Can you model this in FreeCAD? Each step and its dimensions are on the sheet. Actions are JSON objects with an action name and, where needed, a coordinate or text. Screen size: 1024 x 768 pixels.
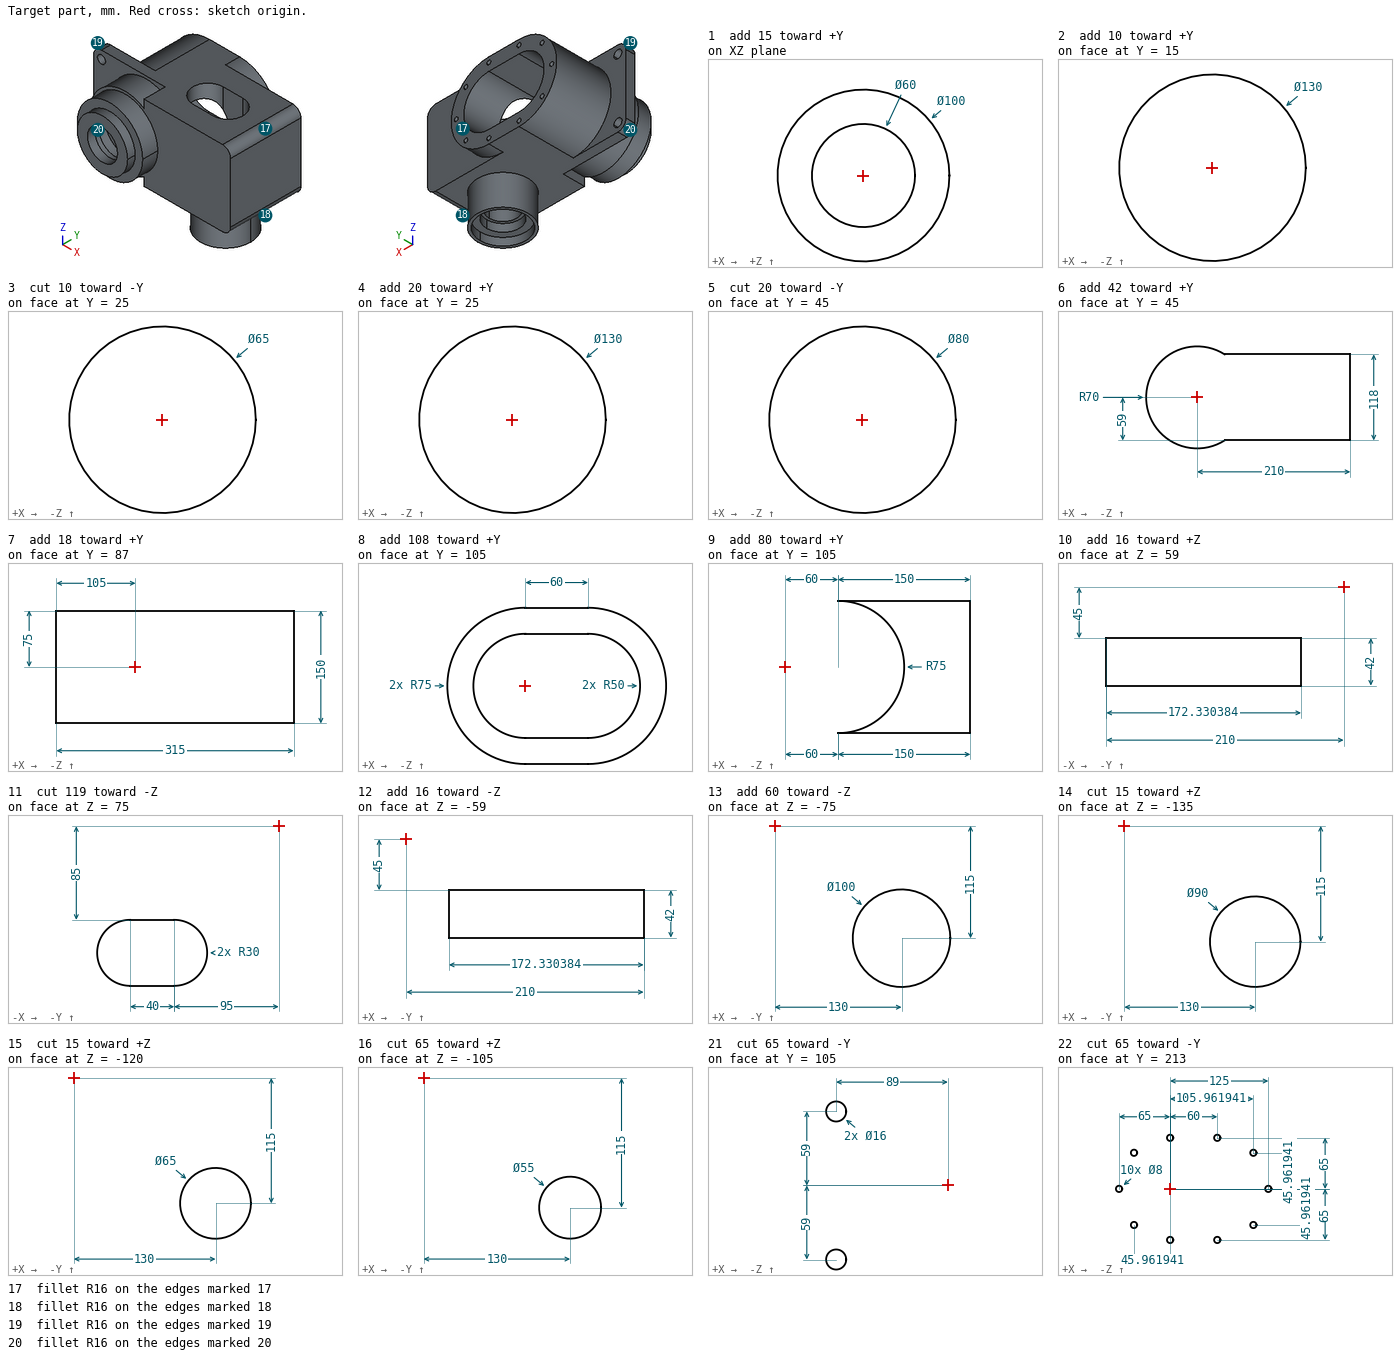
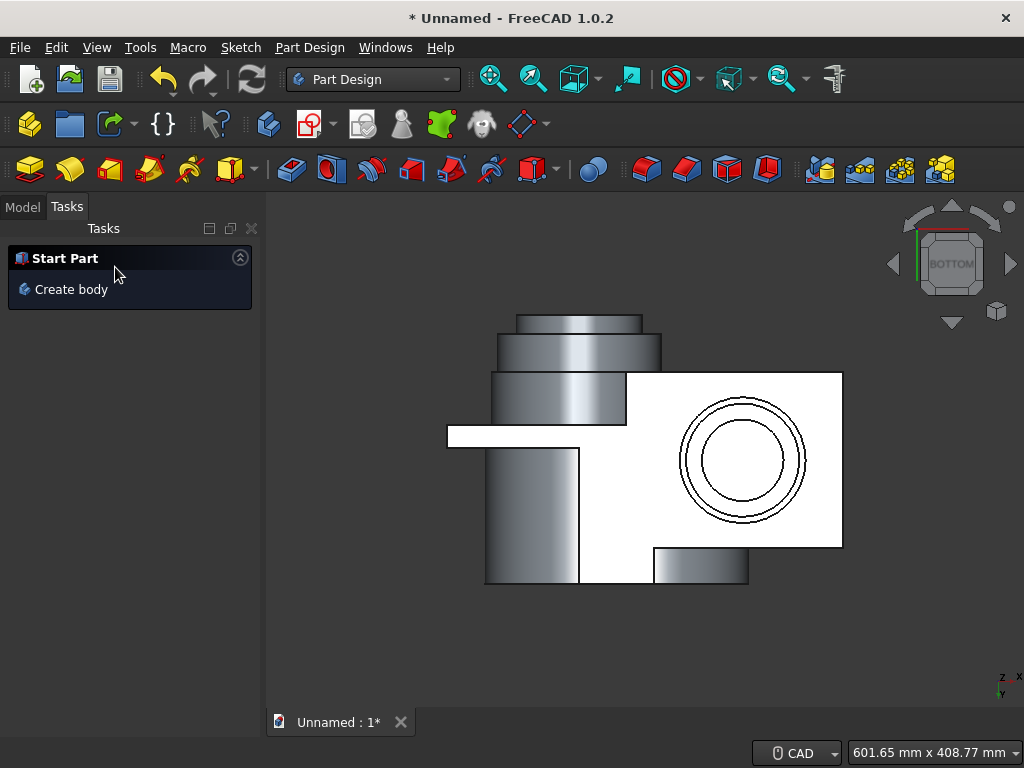
{"action": "left_click", "coordinate": [743, 459]}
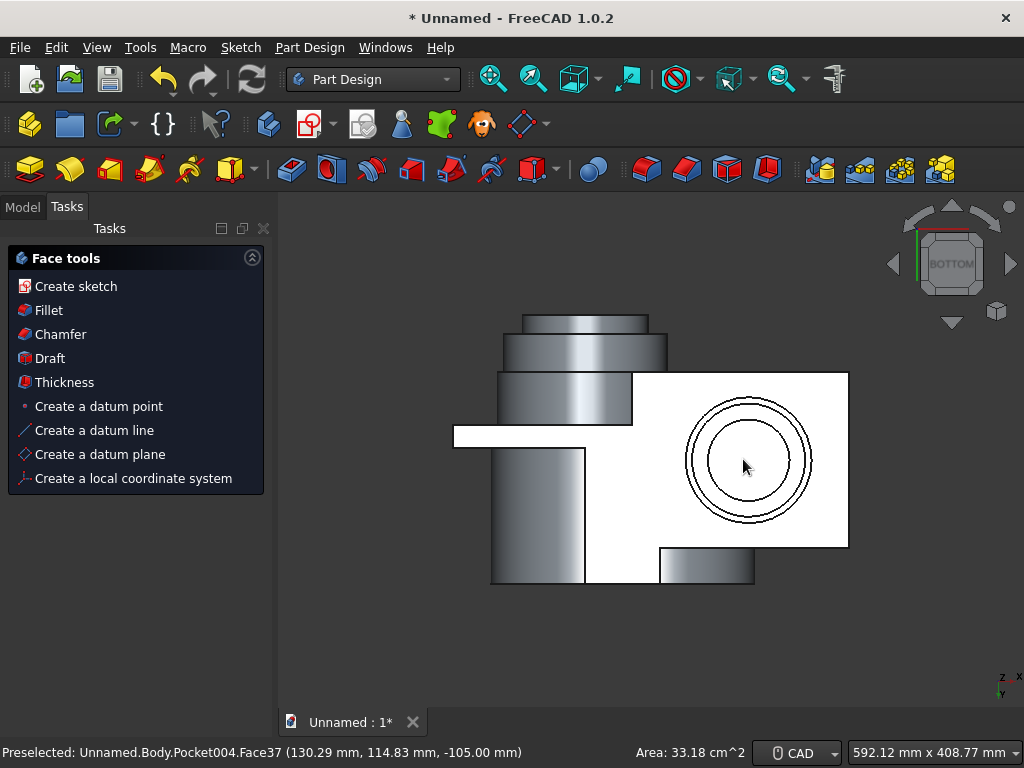
{"action": "left_click", "coordinate": [310, 124]}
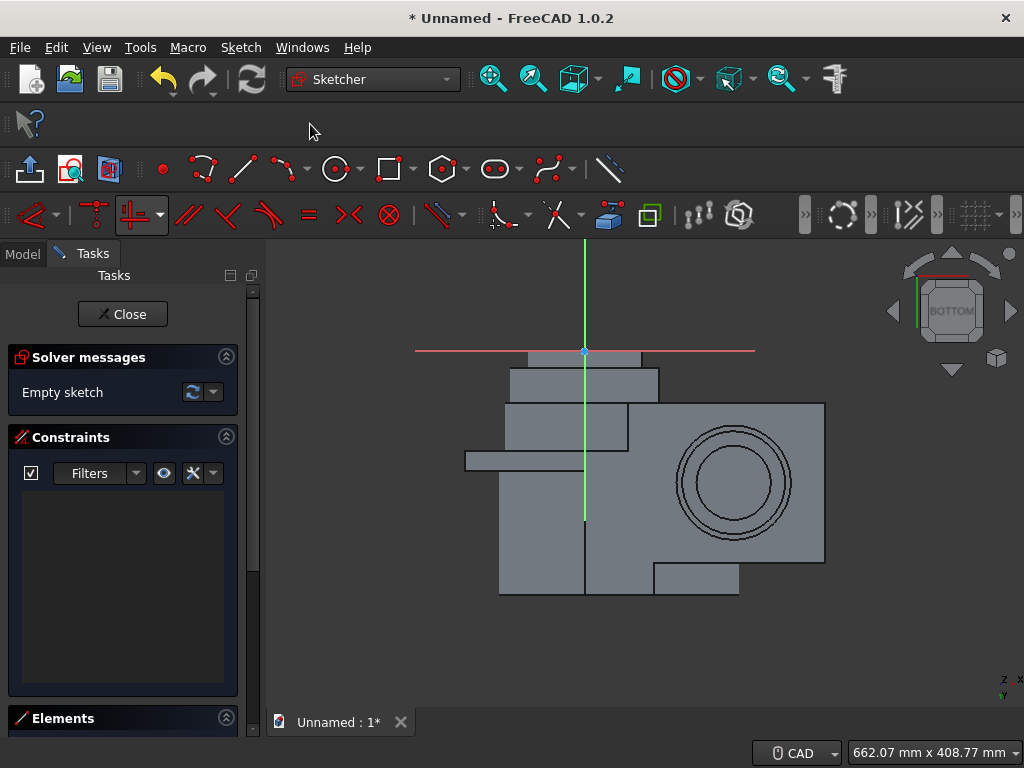
{"action": "left_click", "coordinate": [110, 170]}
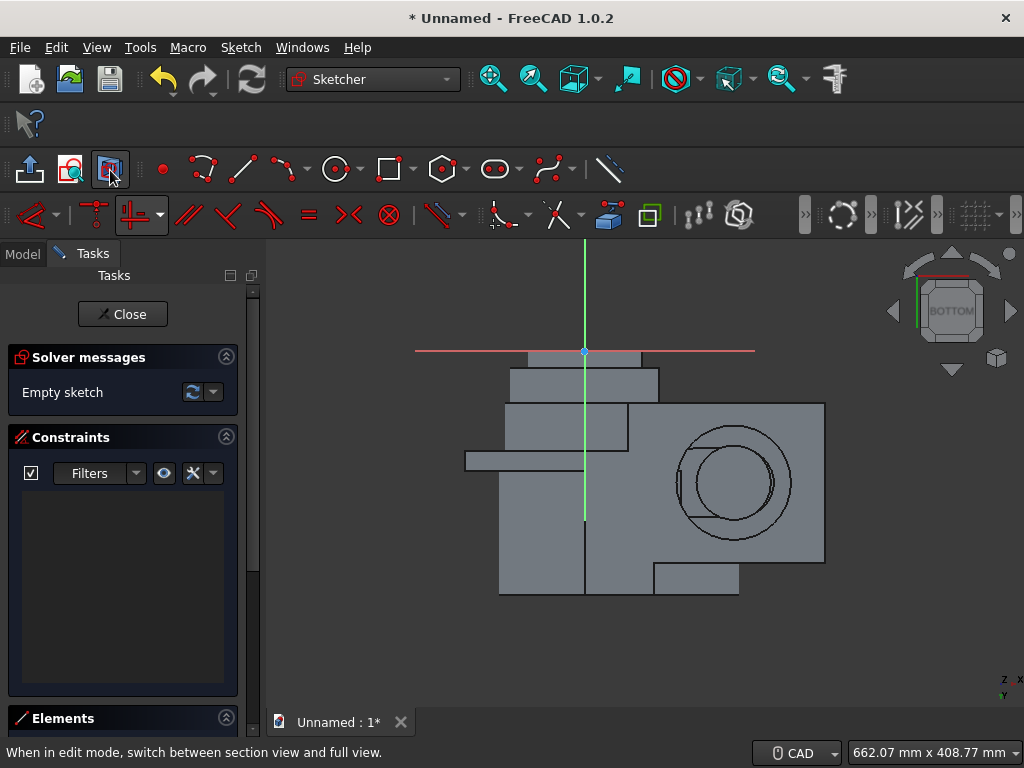
{"action": "scroll", "coordinate": [774, 485], "scroll_direction": "up", "scroll_amount": 8}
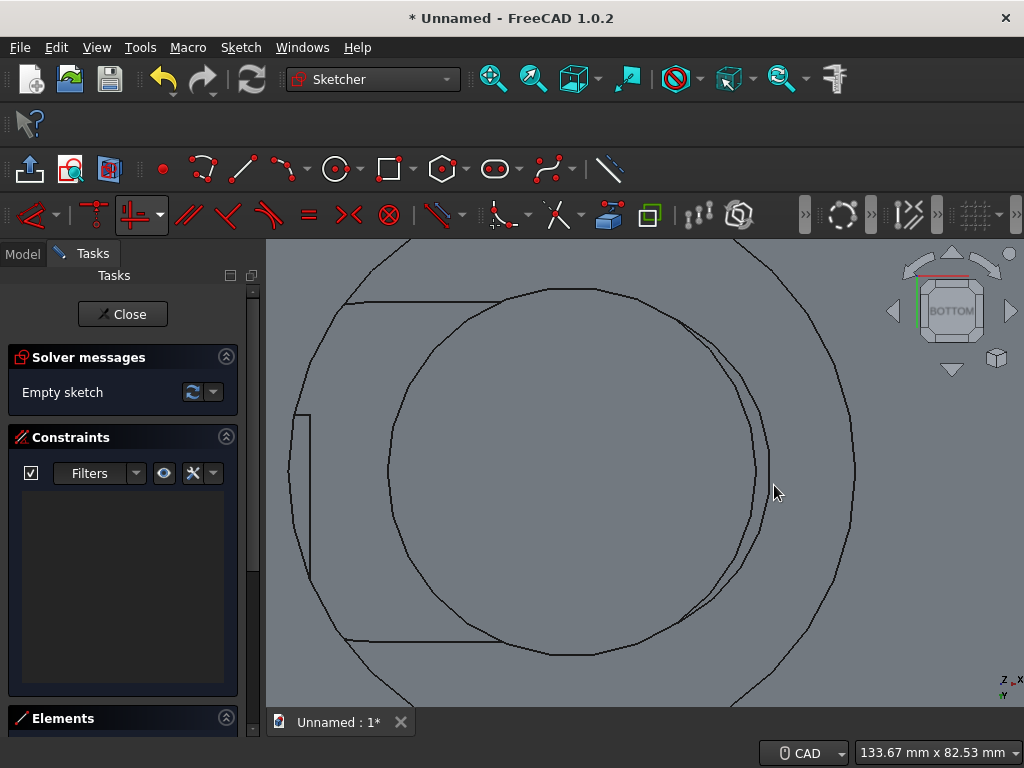
{"action": "left_click", "coordinate": [336, 170]}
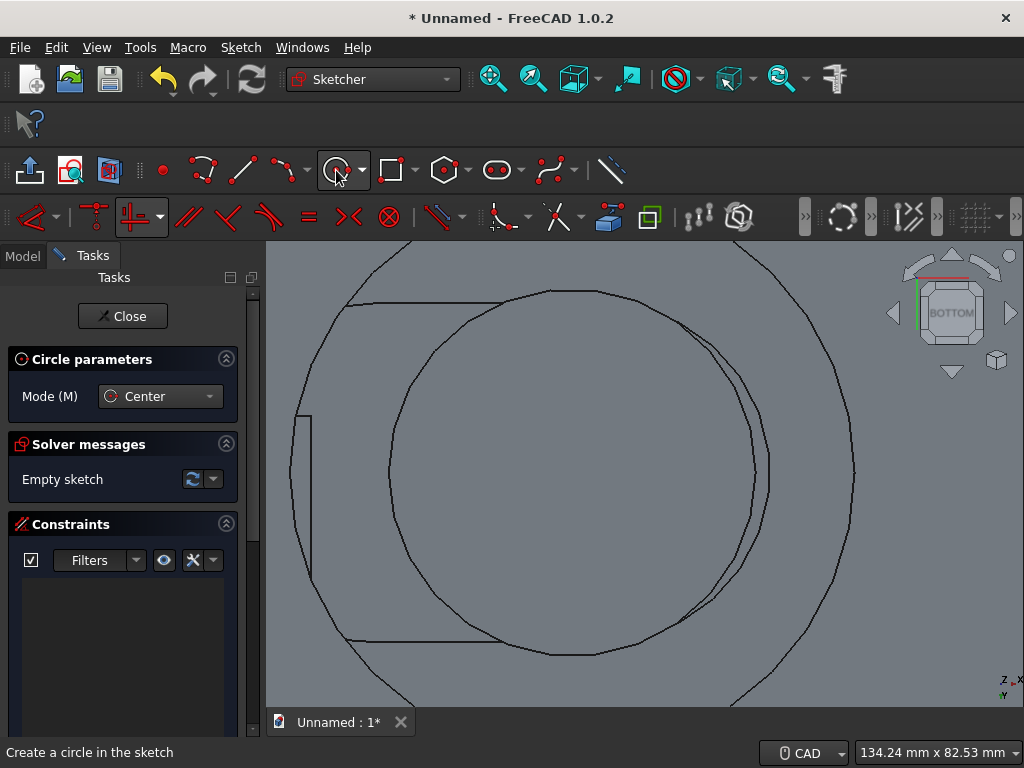
{"action": "left_click", "coordinate": [572, 473]}
{"action": "mouse_move", "coordinate": [682, 363]}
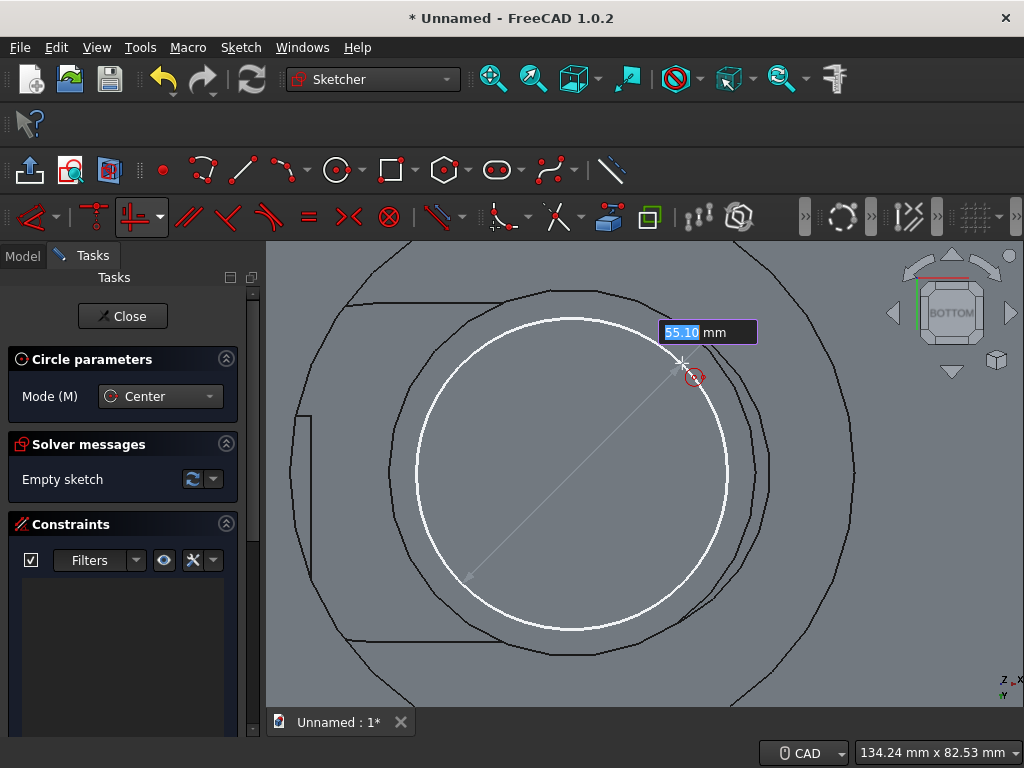
{"action": "type", "text": "55"}
{"action": "key", "text": "Return"}
{"action": "key", "text": "Escape"}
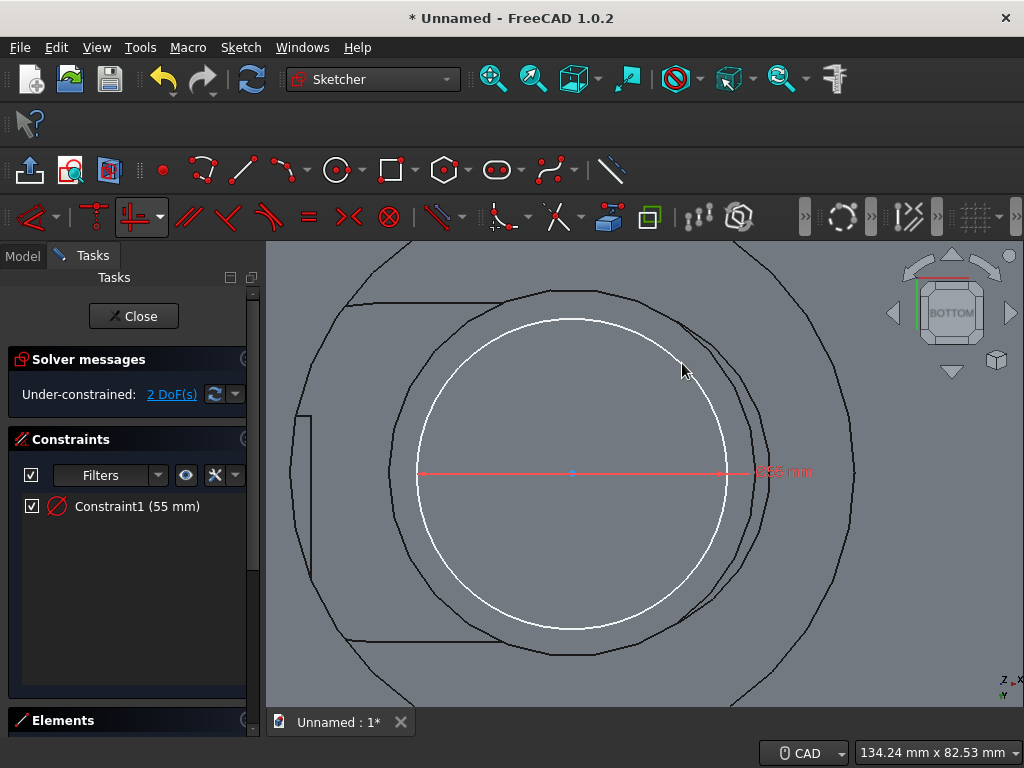
{"action": "left_click", "coordinate": [32, 218]}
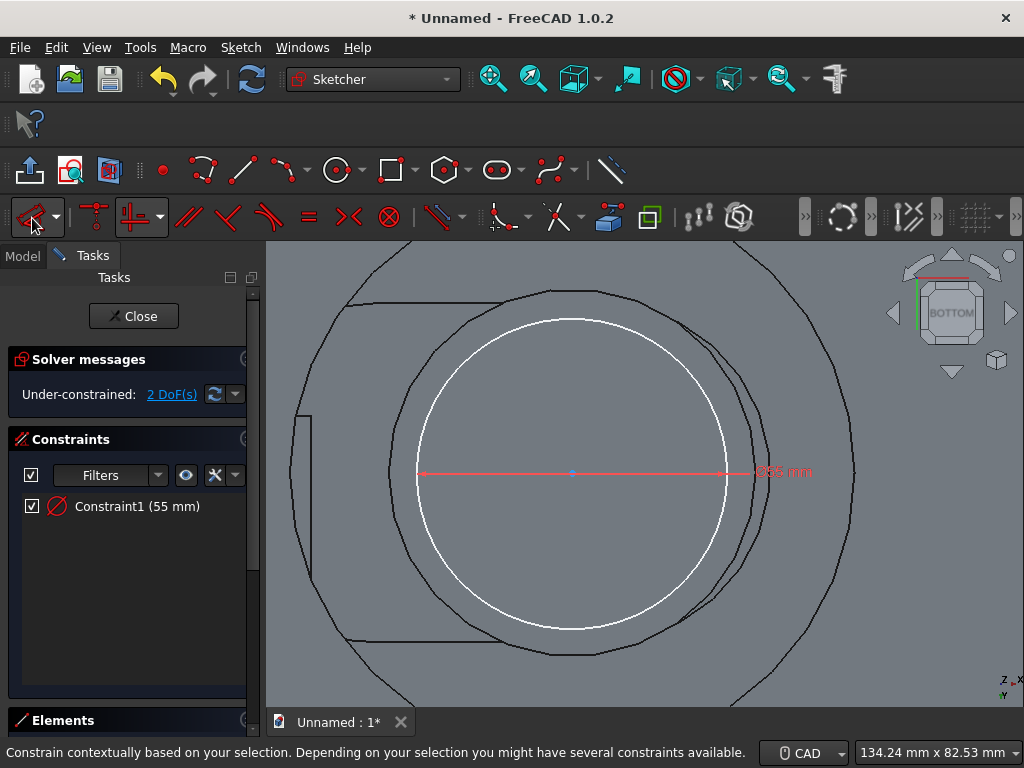
{"action": "left_click", "coordinate": [572, 474]}
{"action": "left_click", "coordinate": [369, 508]}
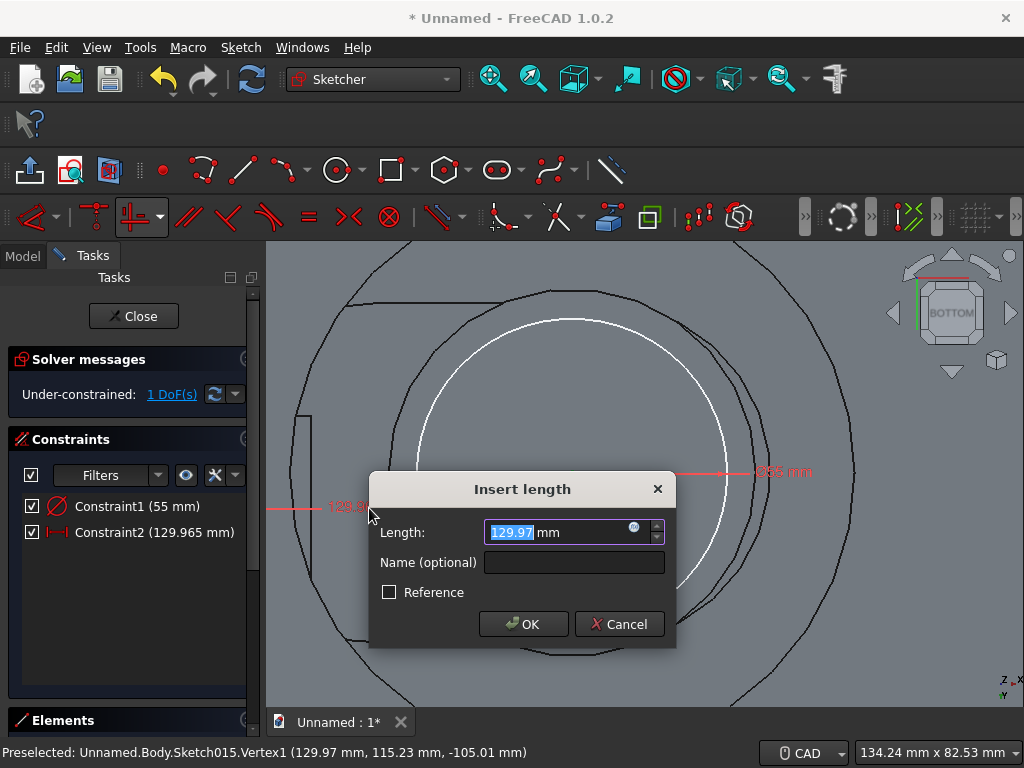
{"action": "type", "text": "130"}
{"action": "key", "text": "Return"}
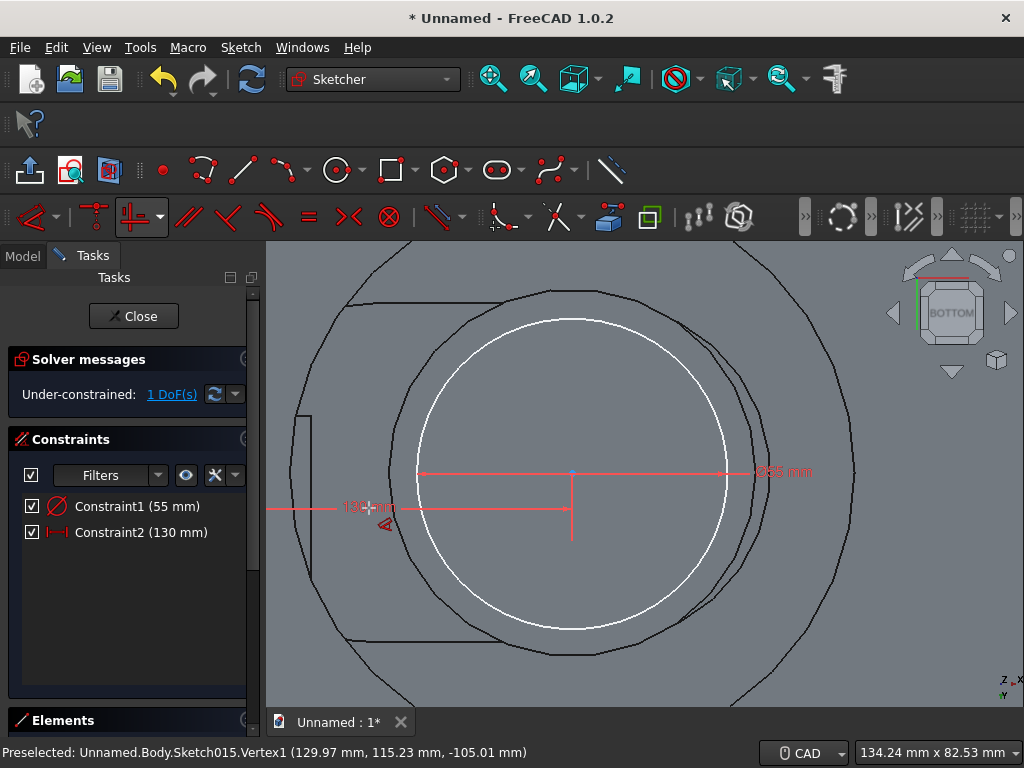
{"action": "left_click", "coordinate": [572, 474]}
{"action": "left_click", "coordinate": [606, 371]}